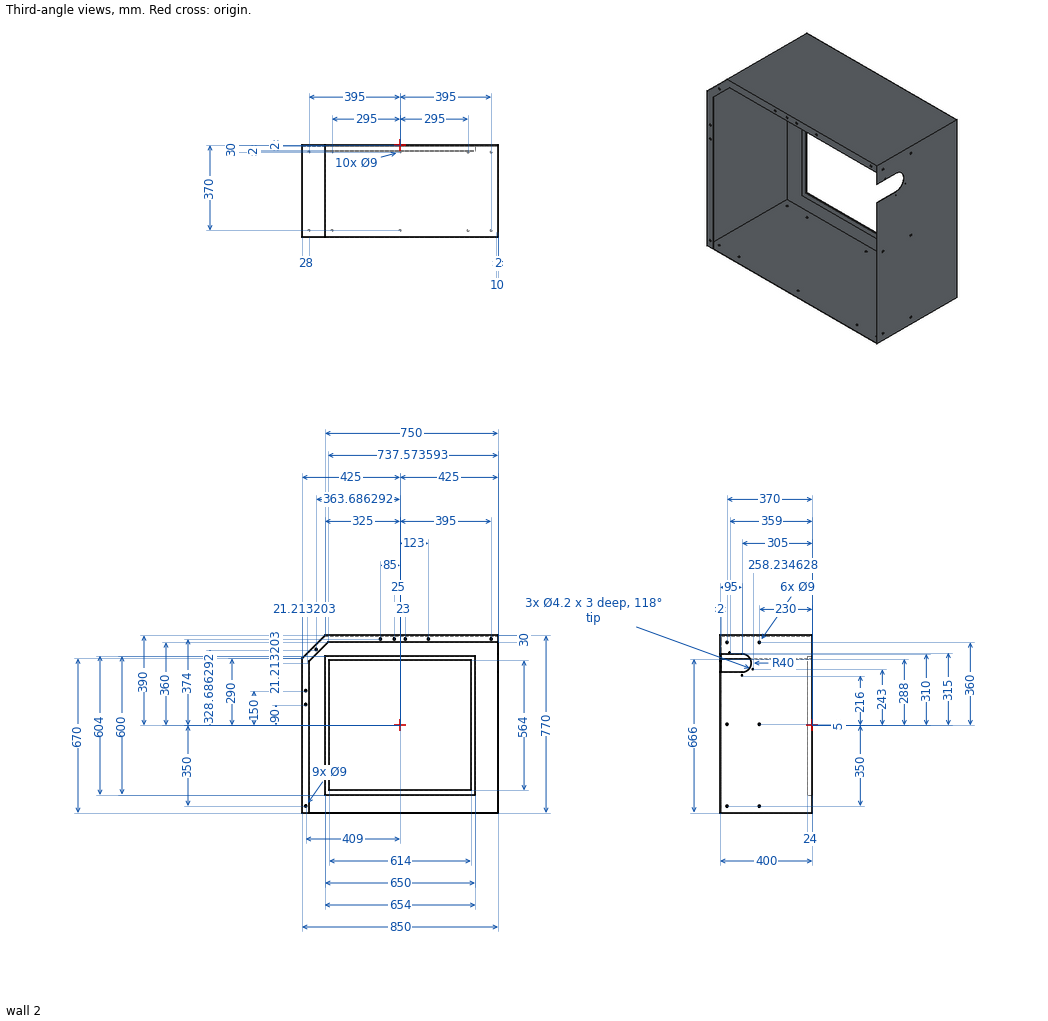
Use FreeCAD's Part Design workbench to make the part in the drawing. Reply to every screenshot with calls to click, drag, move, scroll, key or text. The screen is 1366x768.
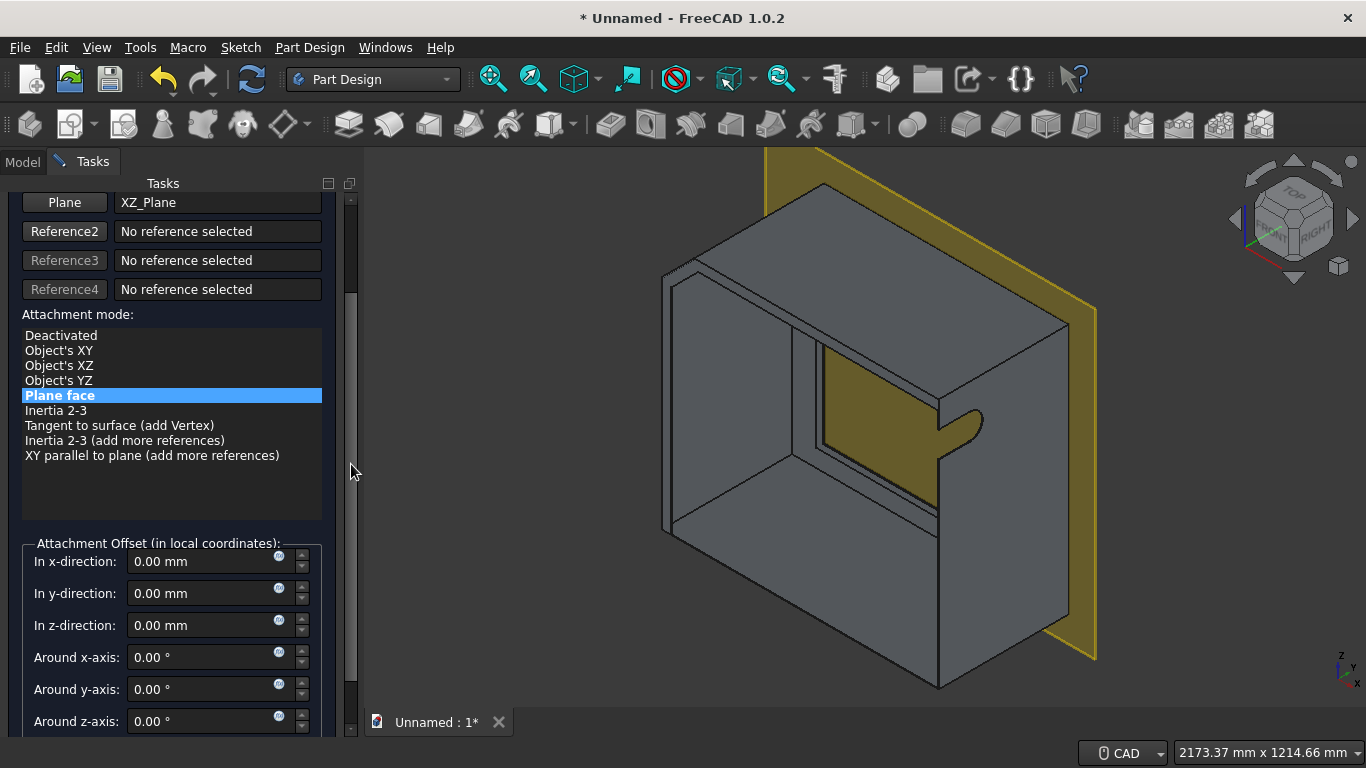
triple_click(210, 625)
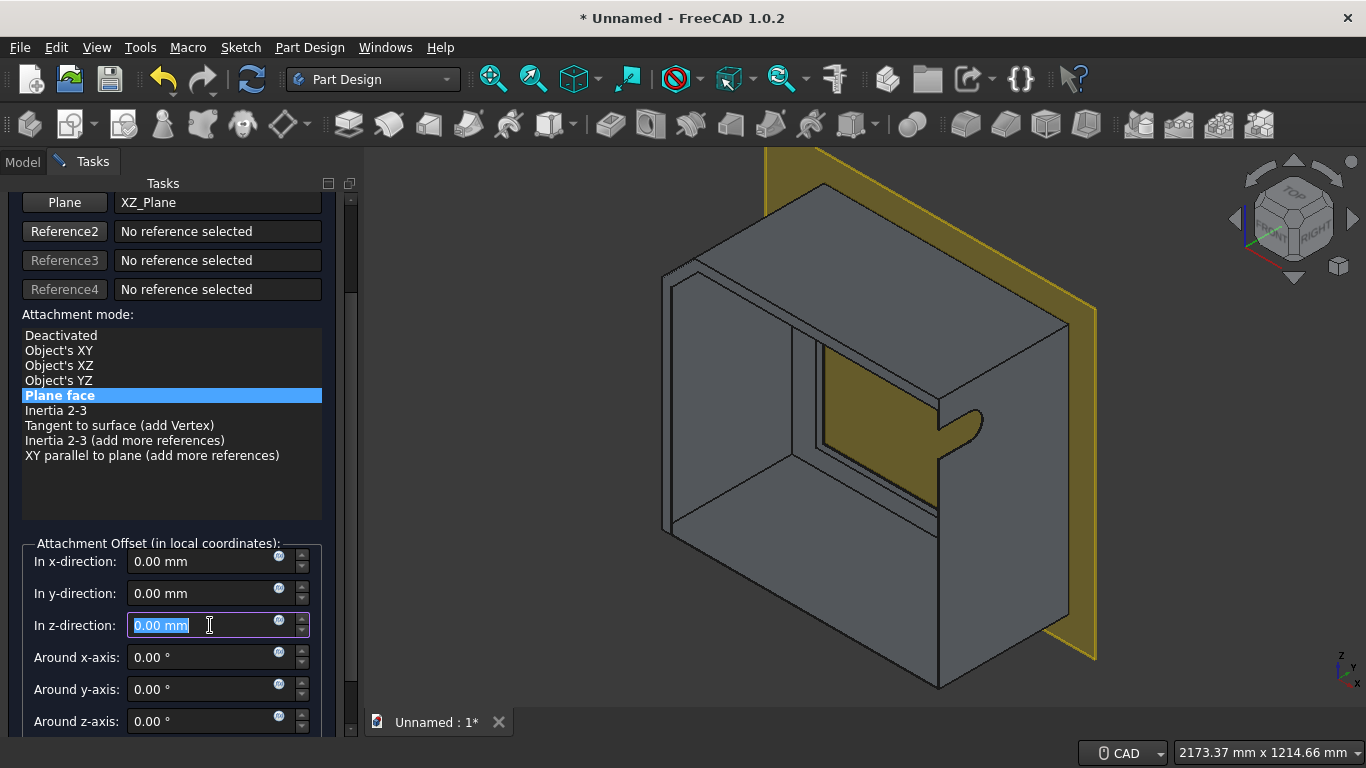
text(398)
key(Tab)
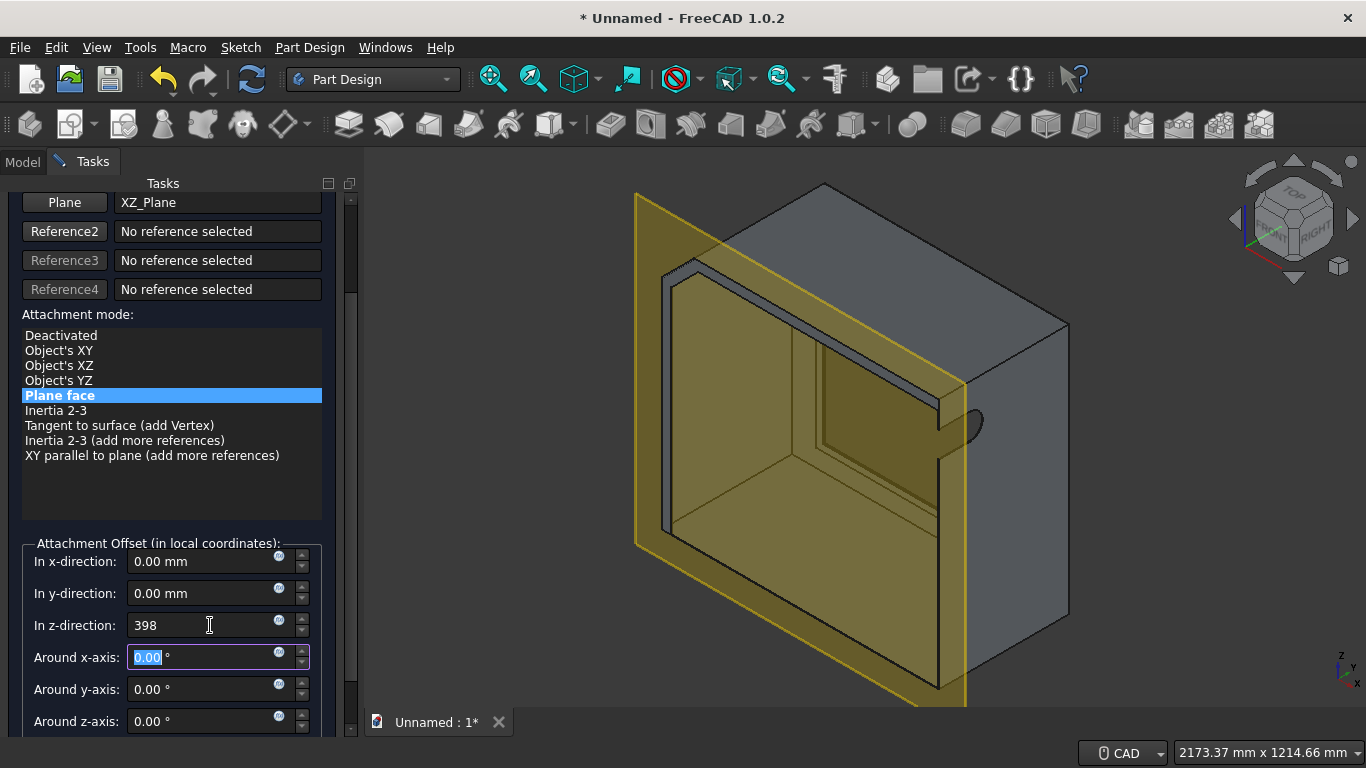
scroll(351, 464, up, 3)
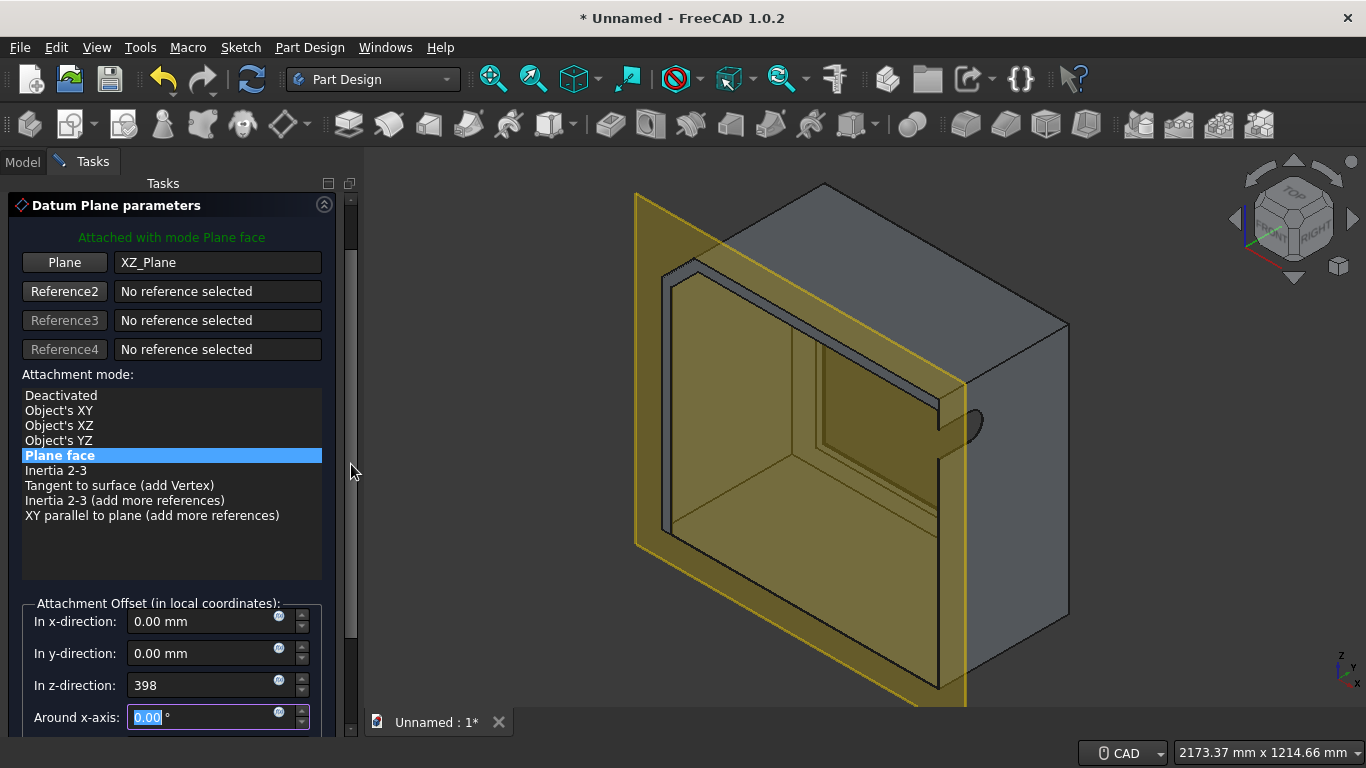
click(124, 222)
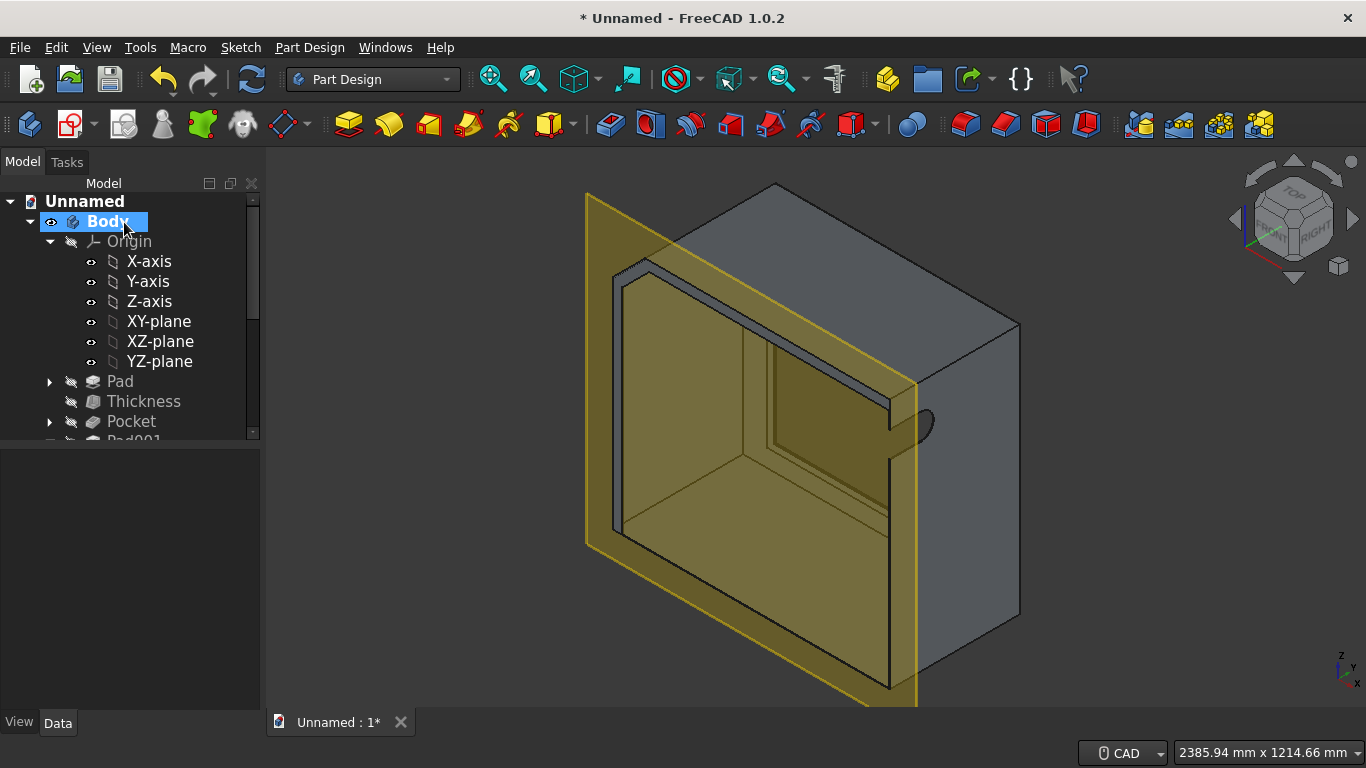
scroll(100, 317, down, 3)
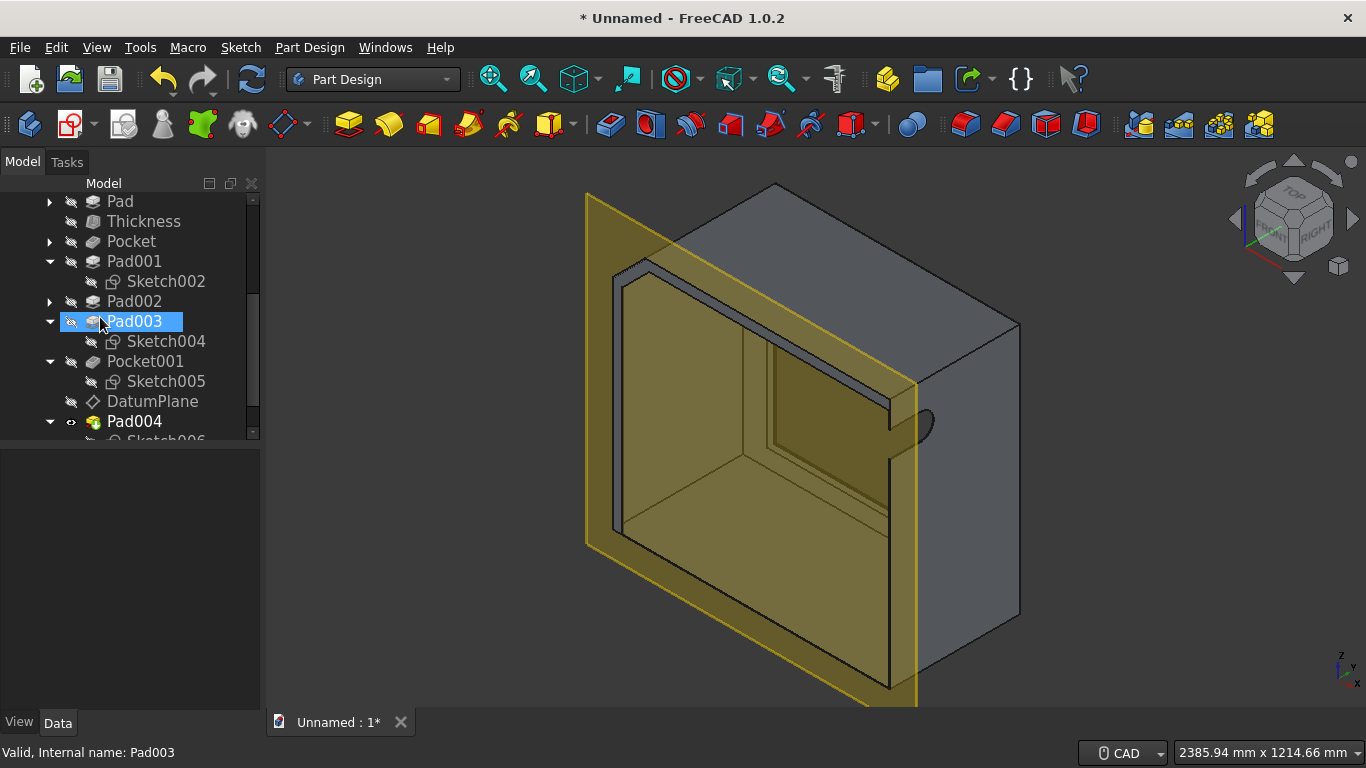
scroll(140, 317, up, 15)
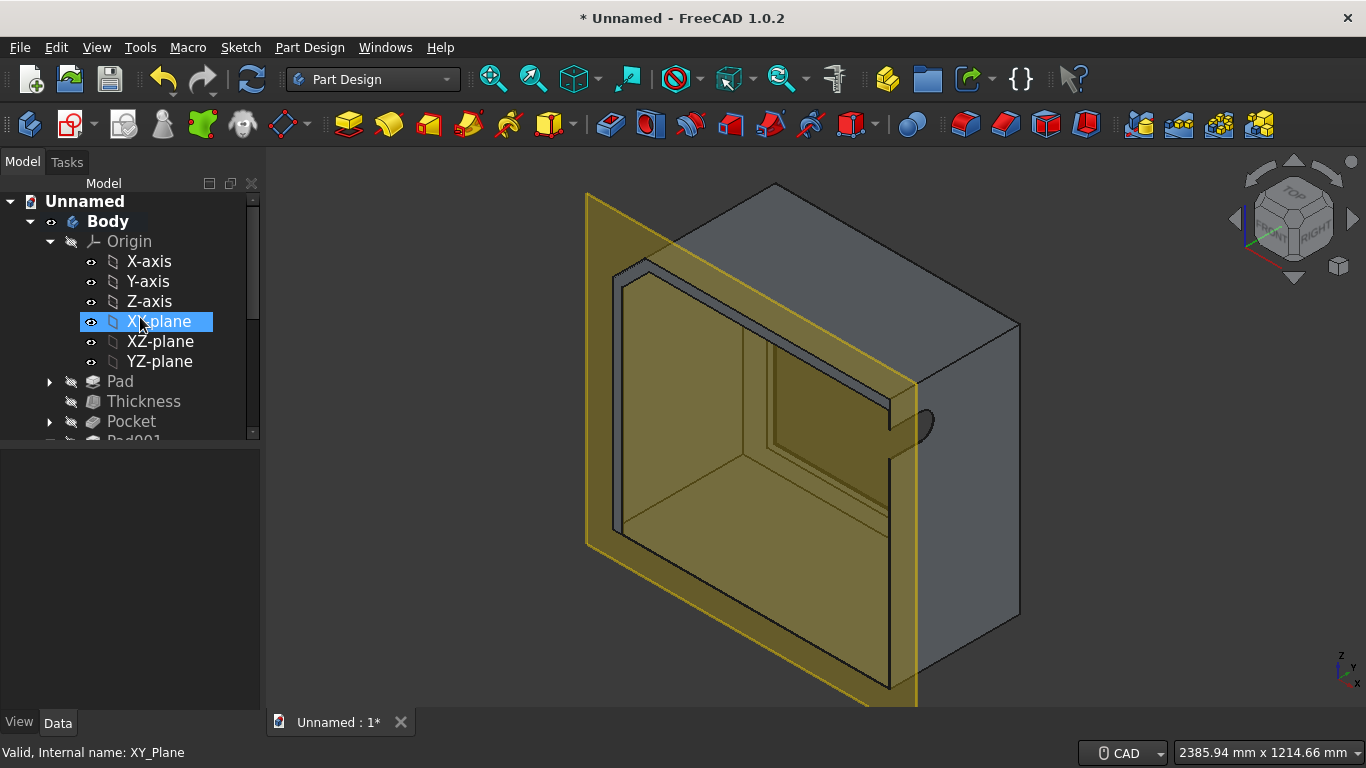
scroll(100, 317, down, 6)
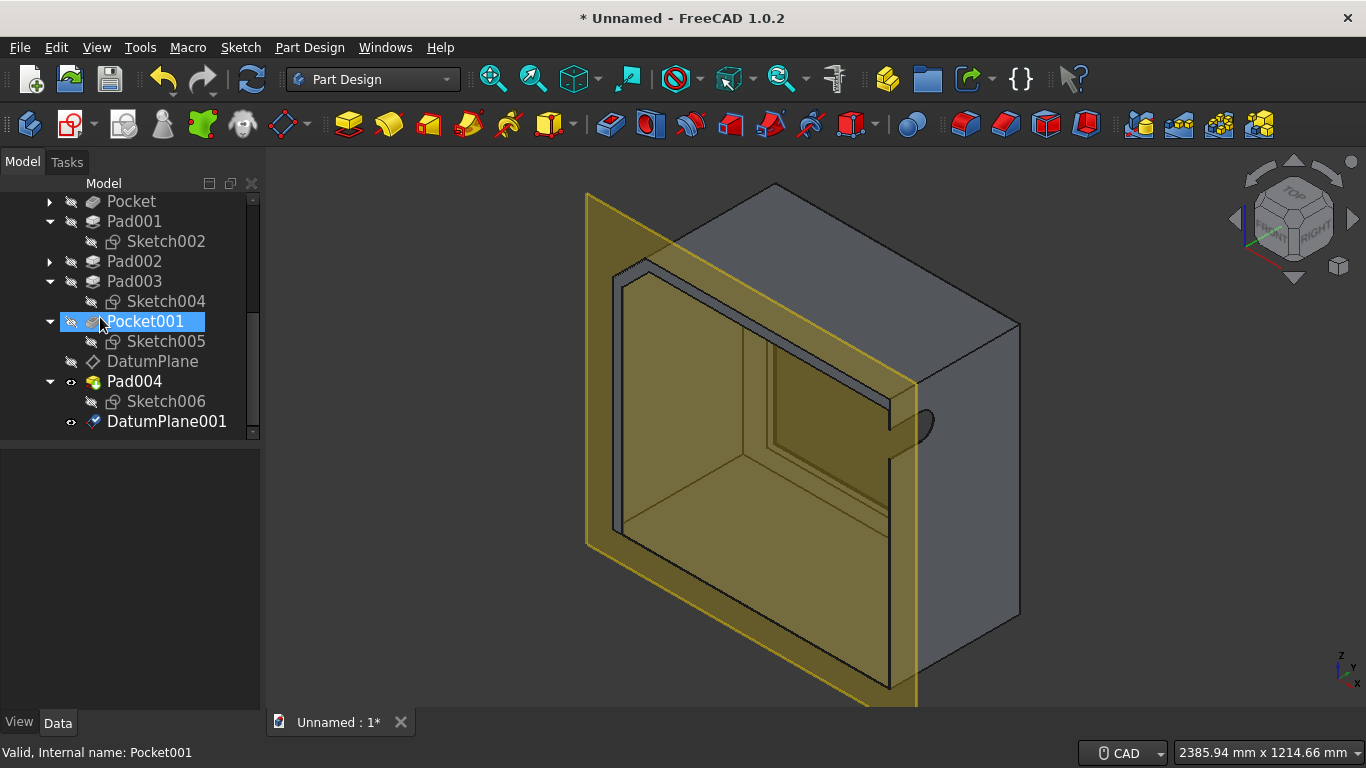
click(116, 422)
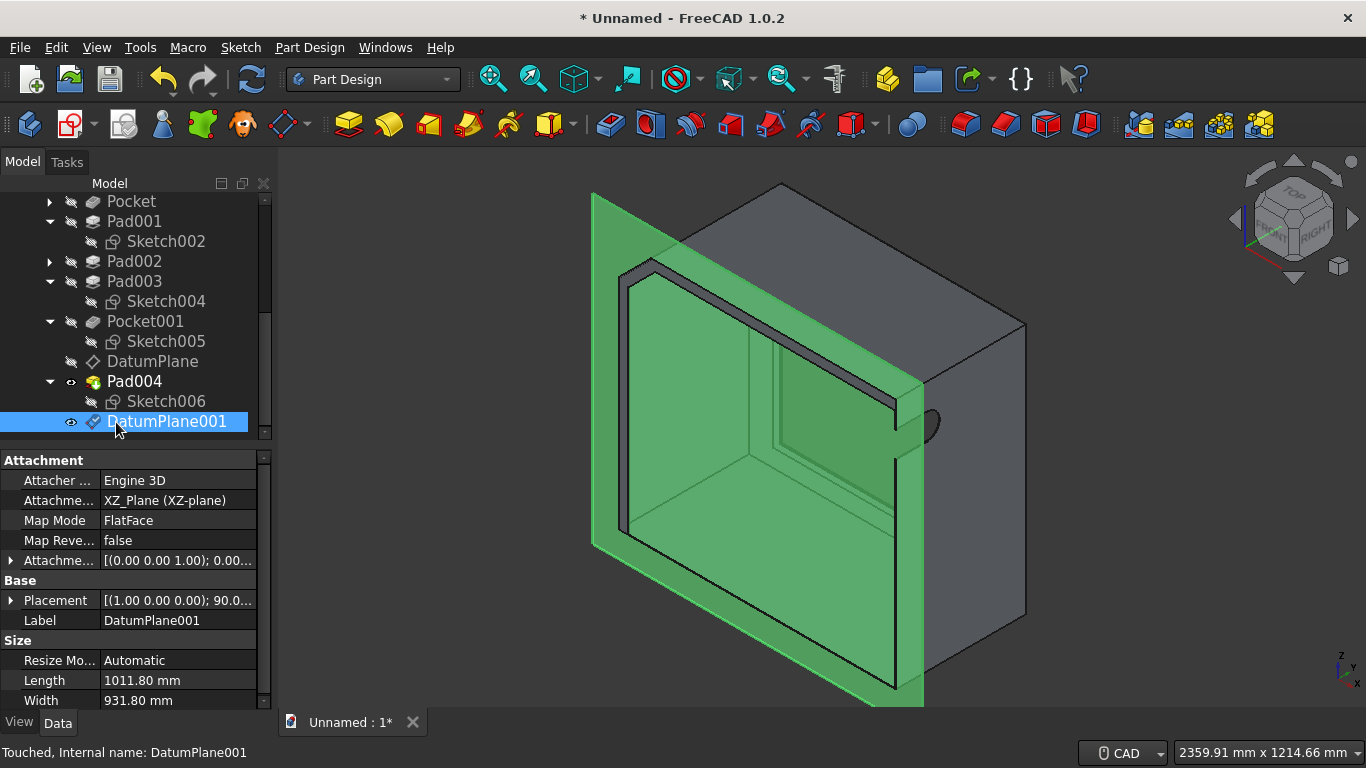
click(70, 124)